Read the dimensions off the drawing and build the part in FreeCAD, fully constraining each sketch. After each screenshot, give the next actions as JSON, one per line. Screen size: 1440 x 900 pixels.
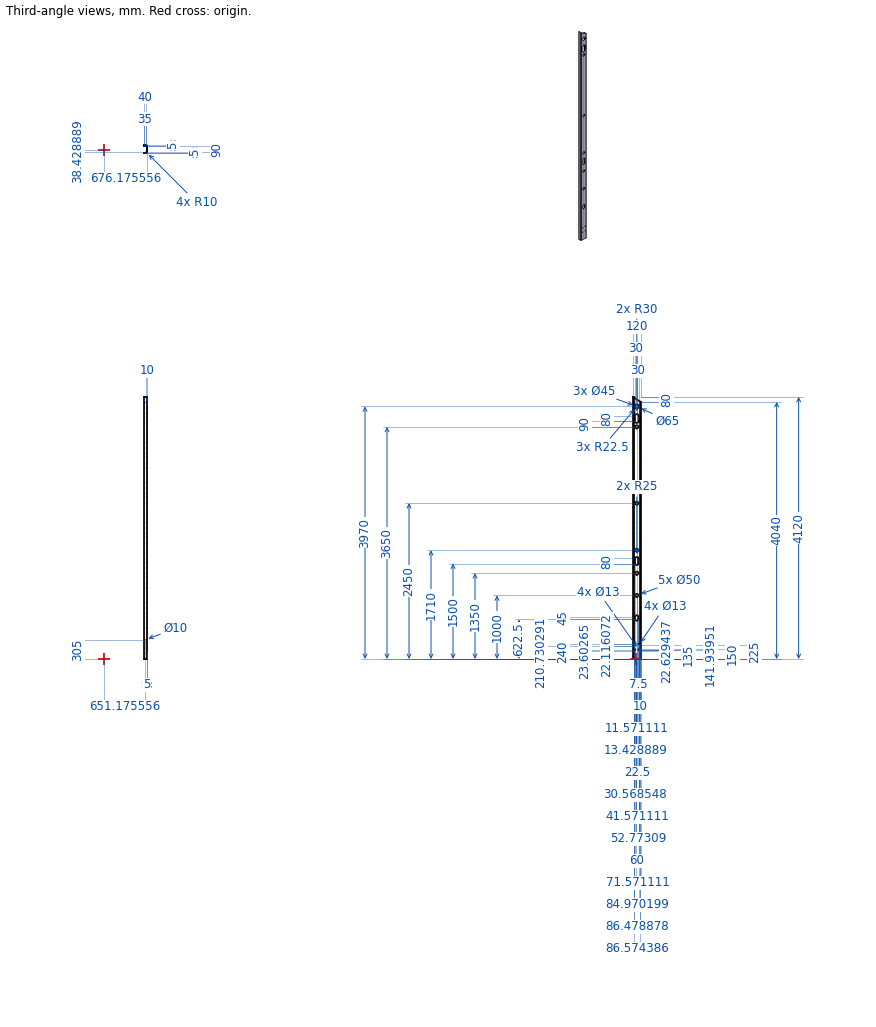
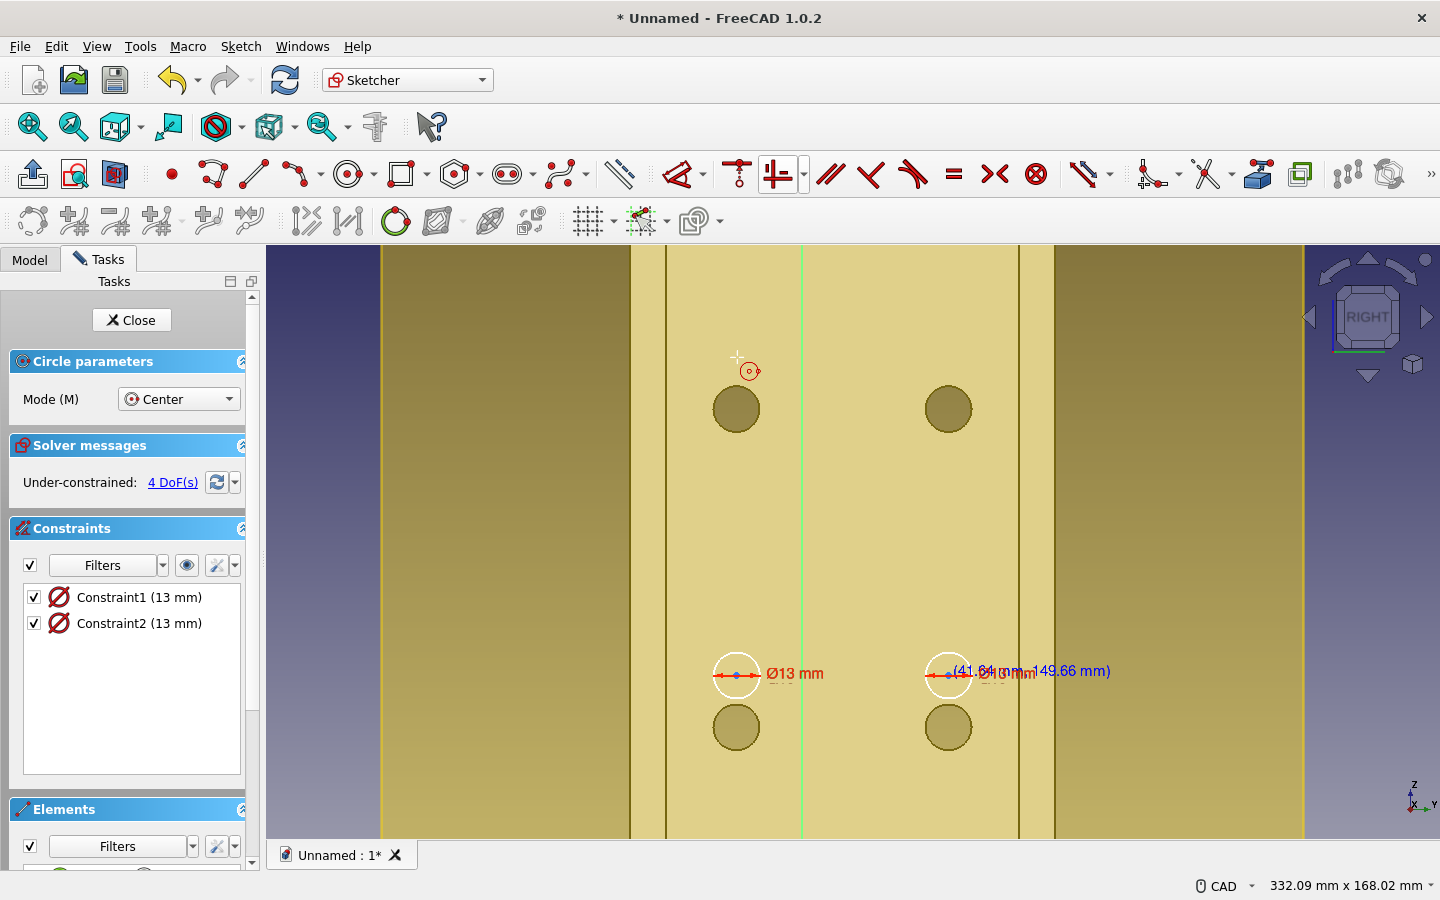
{"action": "left_click", "coordinate": [736, 356]}
{"action": "mouse_move", "coordinate": [753, 340]}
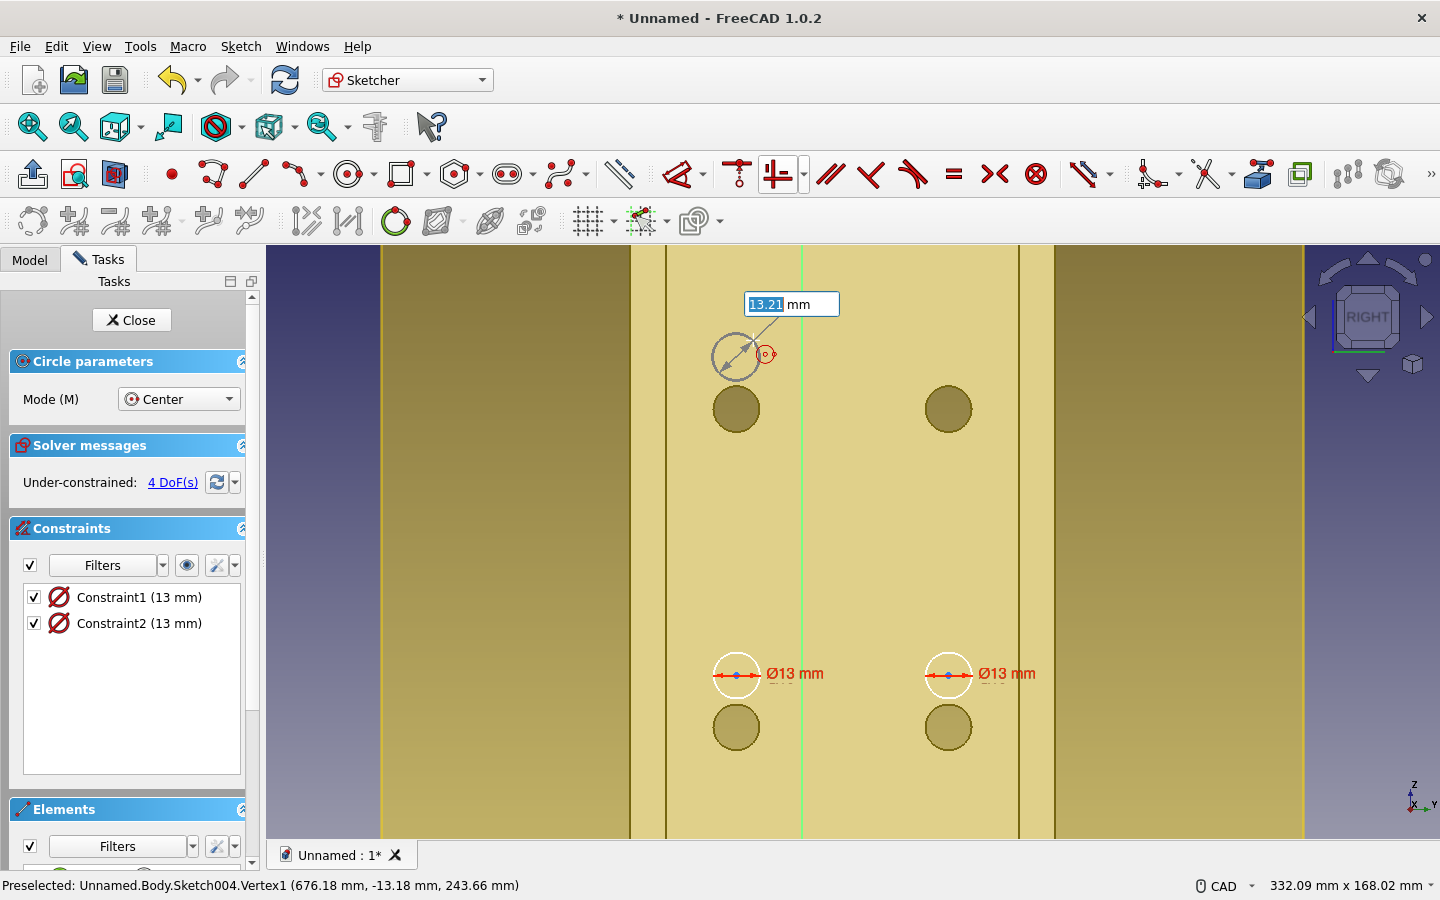
{"action": "type", "text": "13"}
{"action": "key", "text": "Return"}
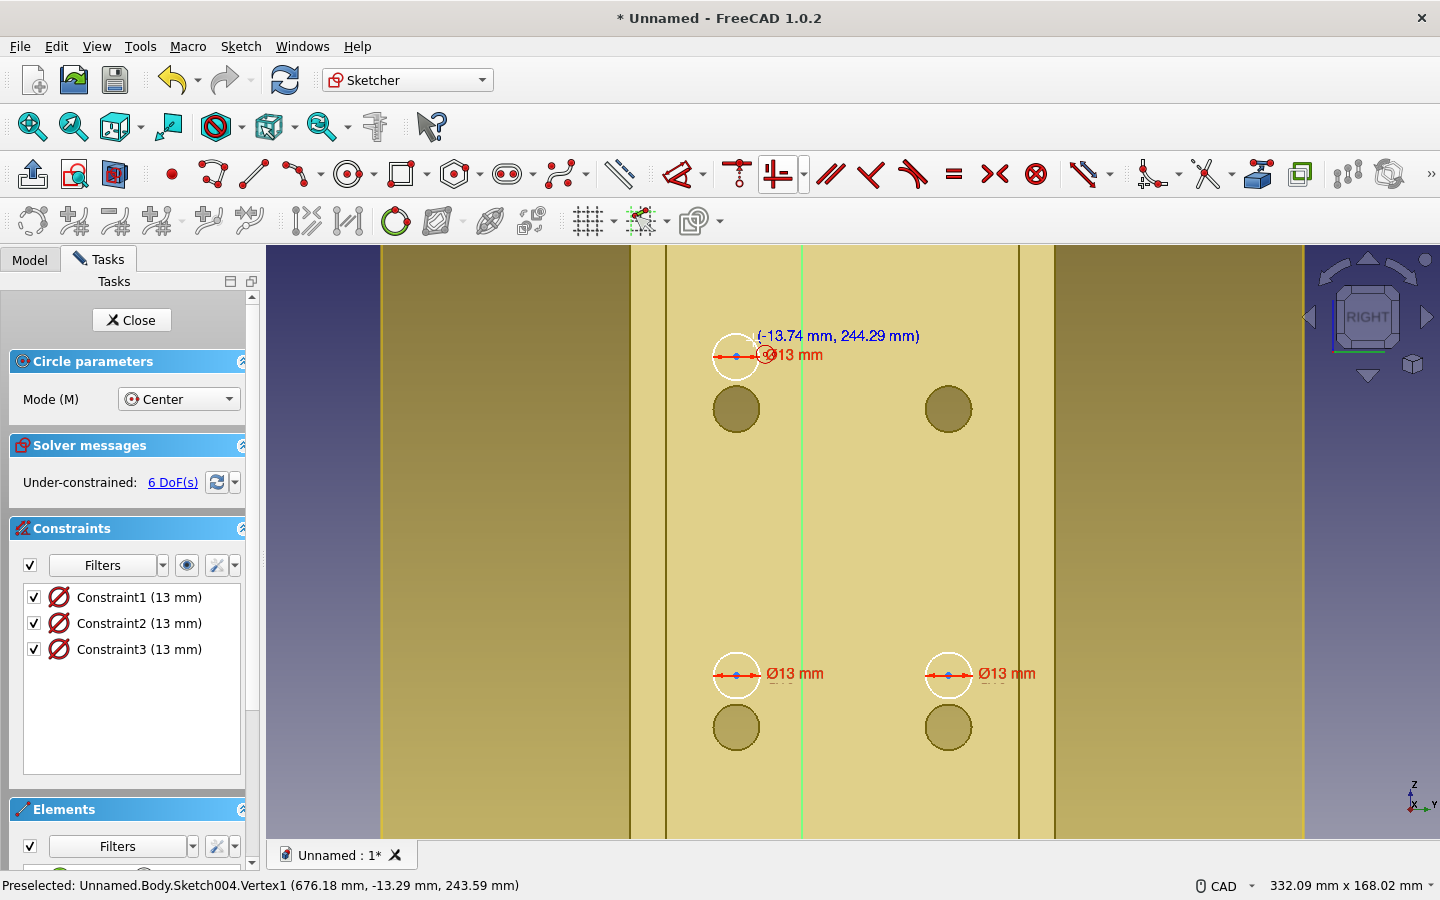
{"action": "left_click", "coordinate": [949, 356]}
{"action": "mouse_move", "coordinate": [965, 340]}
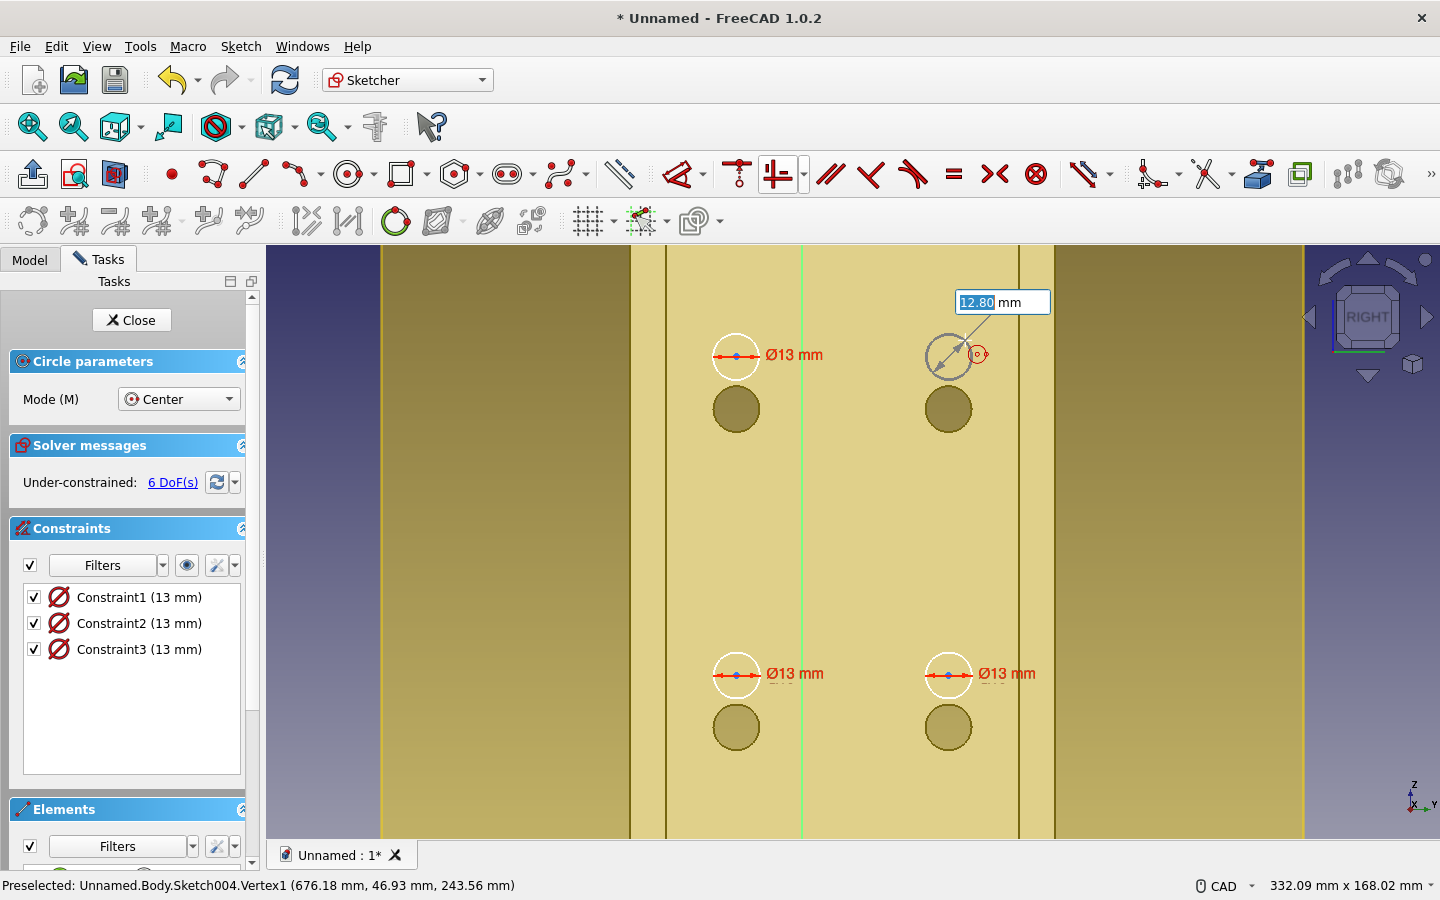
{"action": "type", "text": "13"}
{"action": "key", "text": "Return"}
{"action": "key", "text": "Escape"}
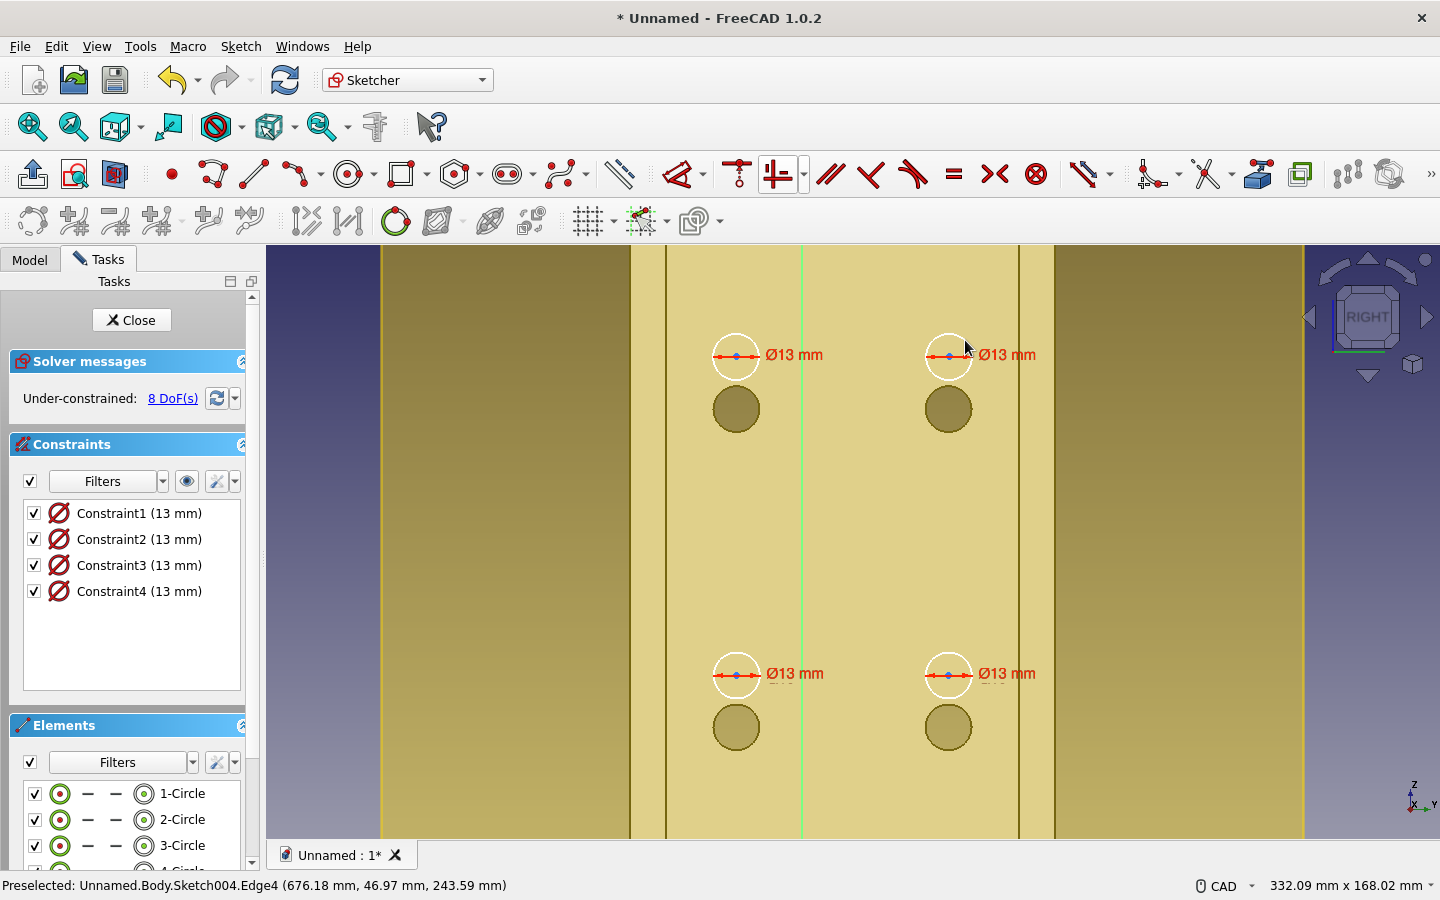
{"action": "left_click", "coordinate": [949, 676]}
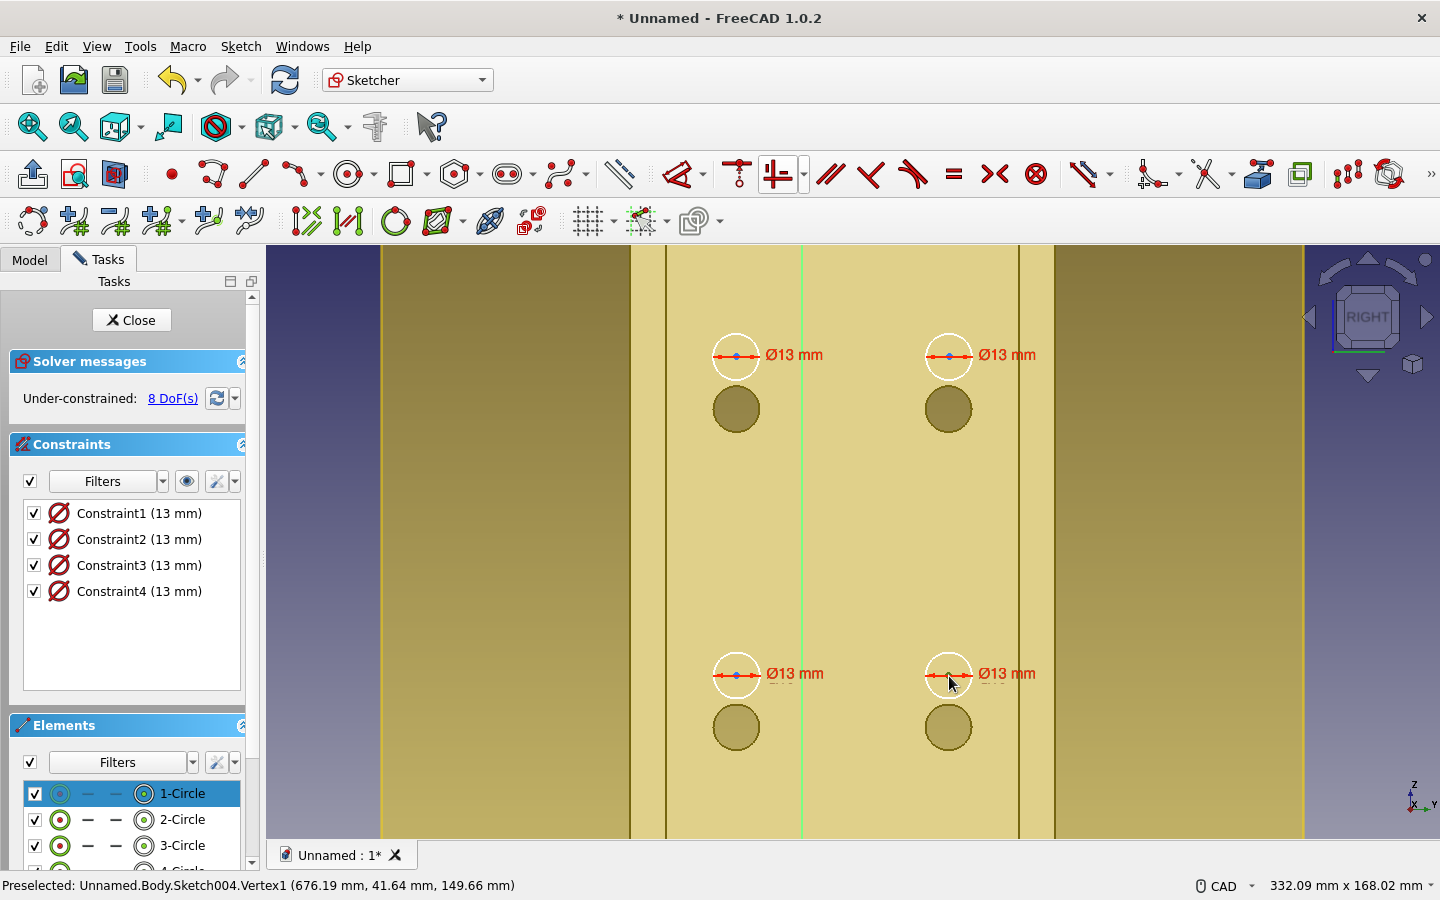
{"action": "left_click", "coordinate": [737, 676]}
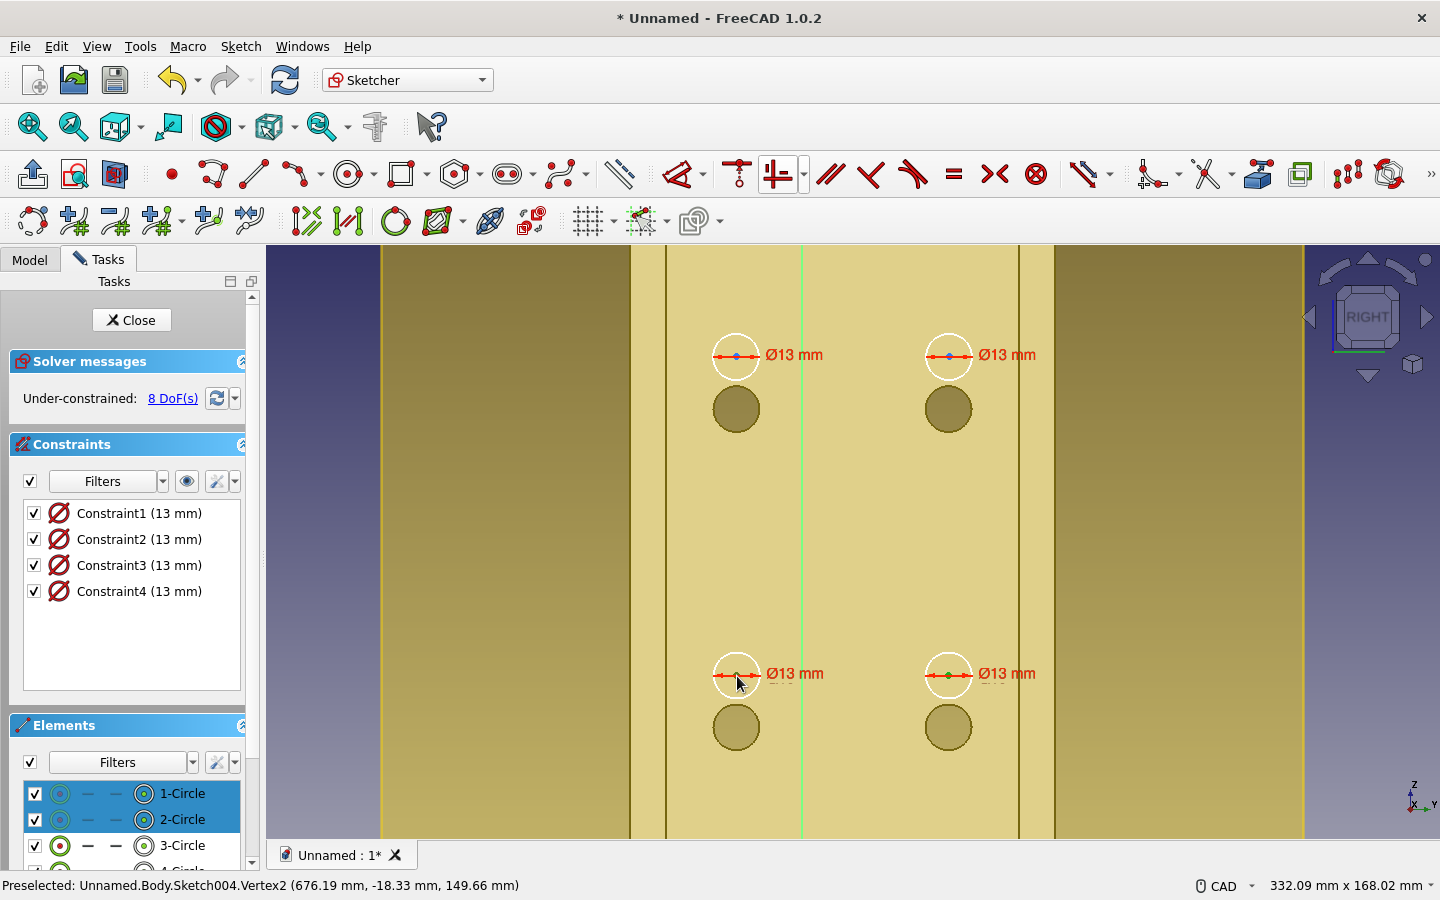
{"action": "key", "text": "h"}